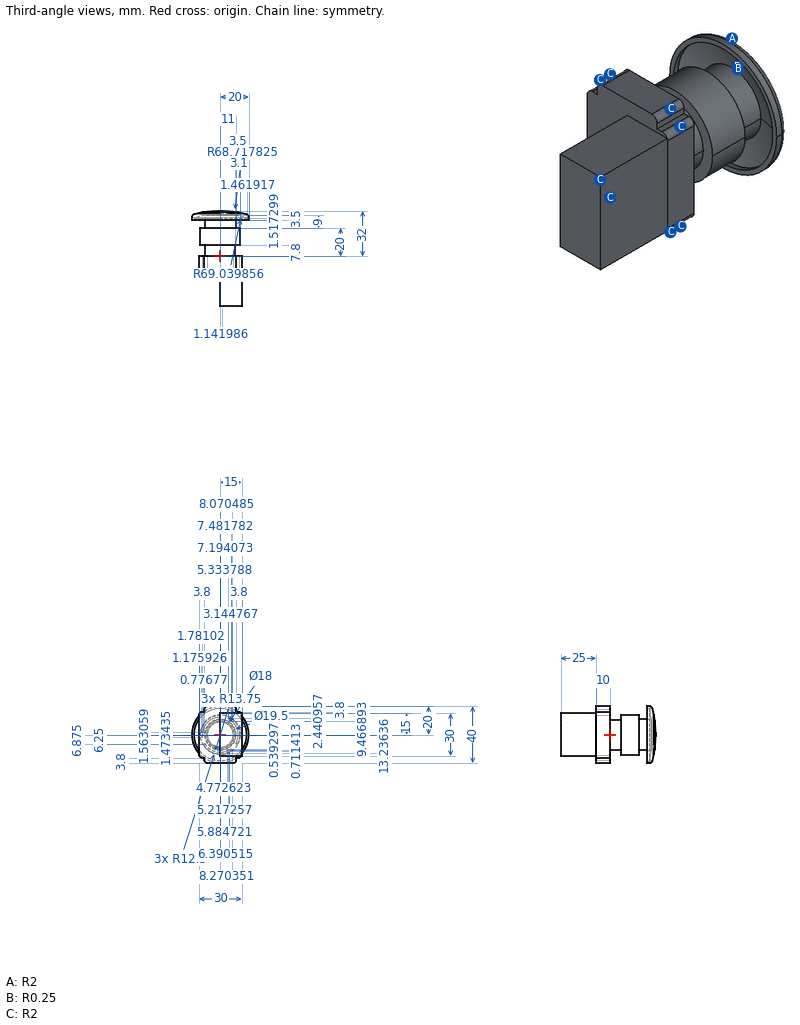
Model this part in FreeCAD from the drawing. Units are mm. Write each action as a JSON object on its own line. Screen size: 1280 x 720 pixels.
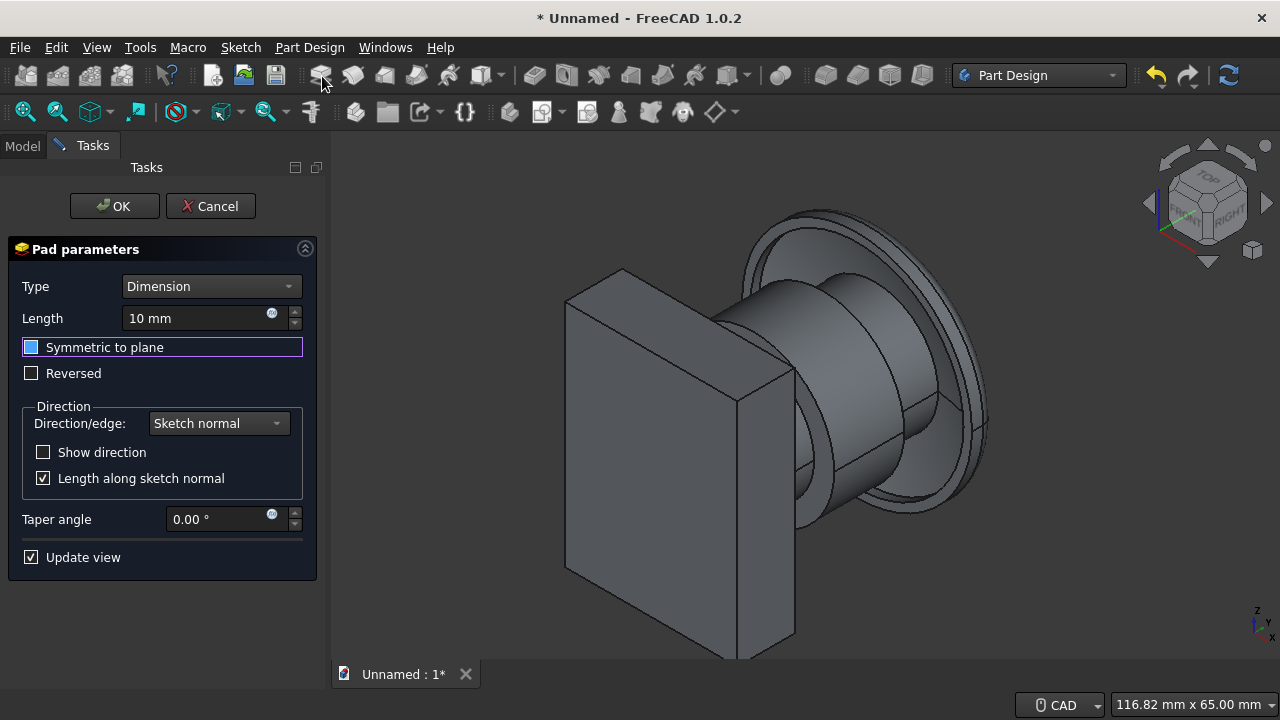
{"action": "left_click", "coordinate": [115, 206]}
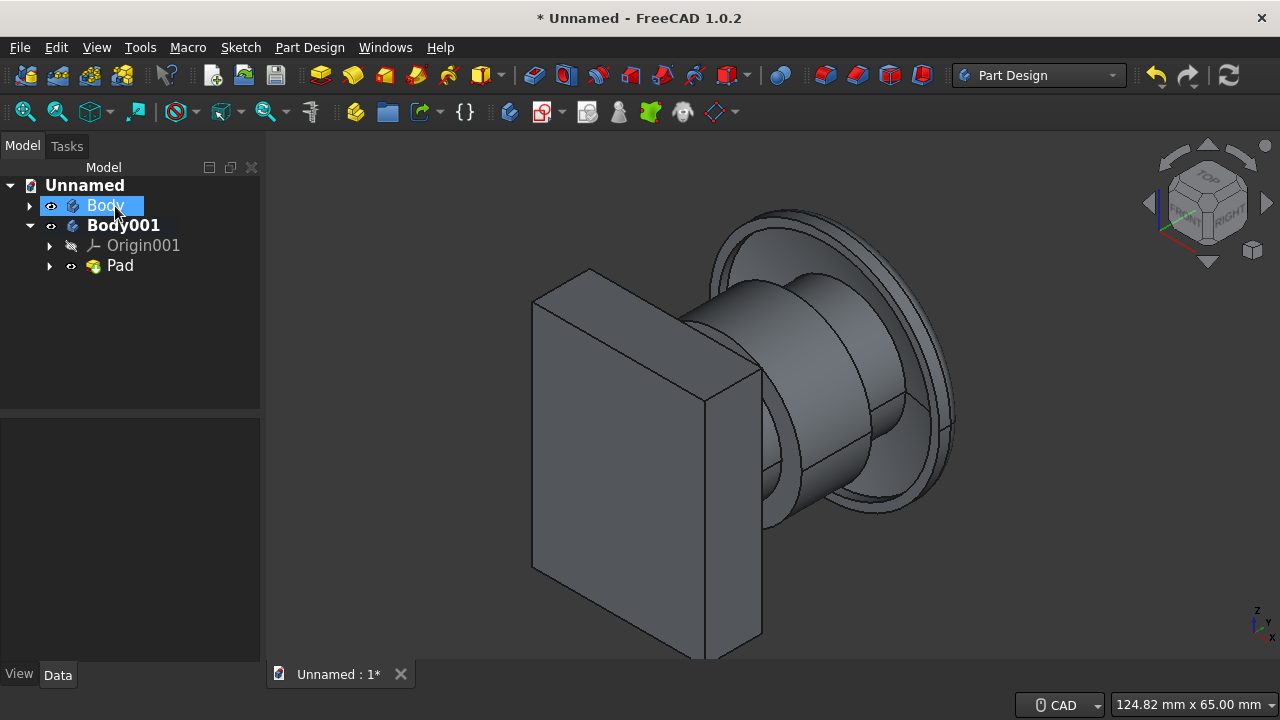
{"action": "left_click", "coordinate": [26, 112]}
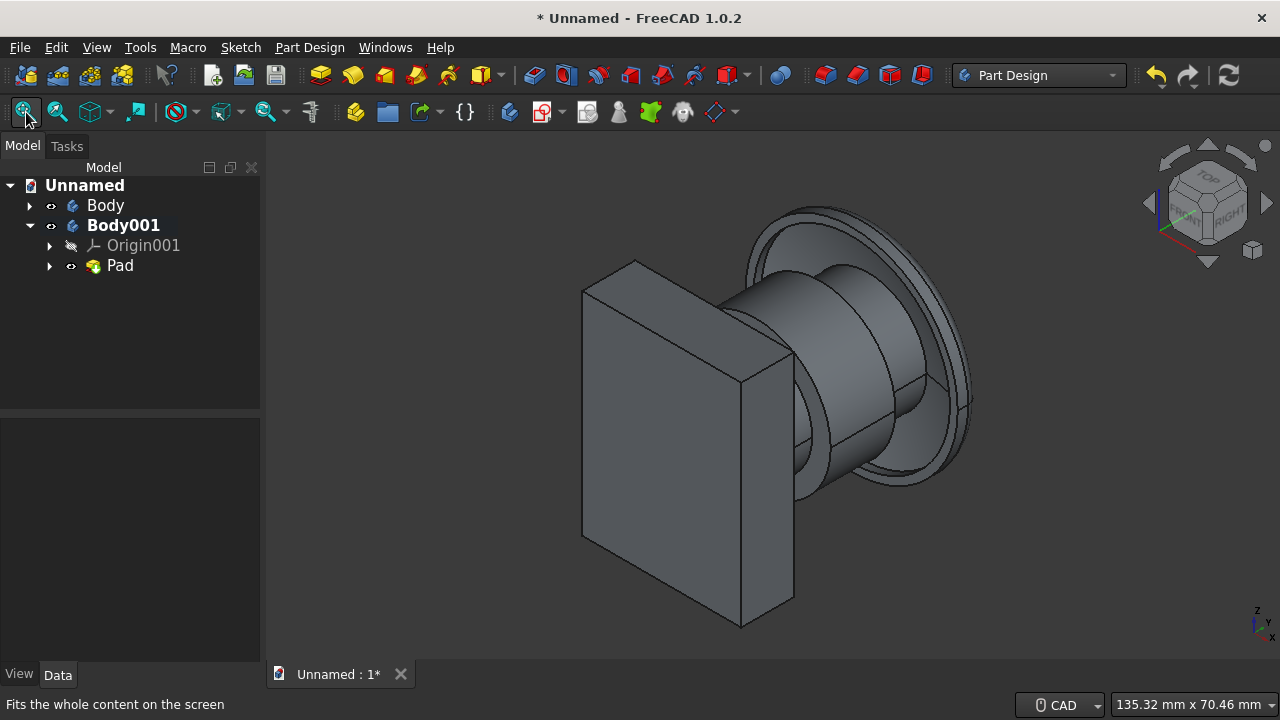
{"action": "left_click", "coordinate": [542, 112]}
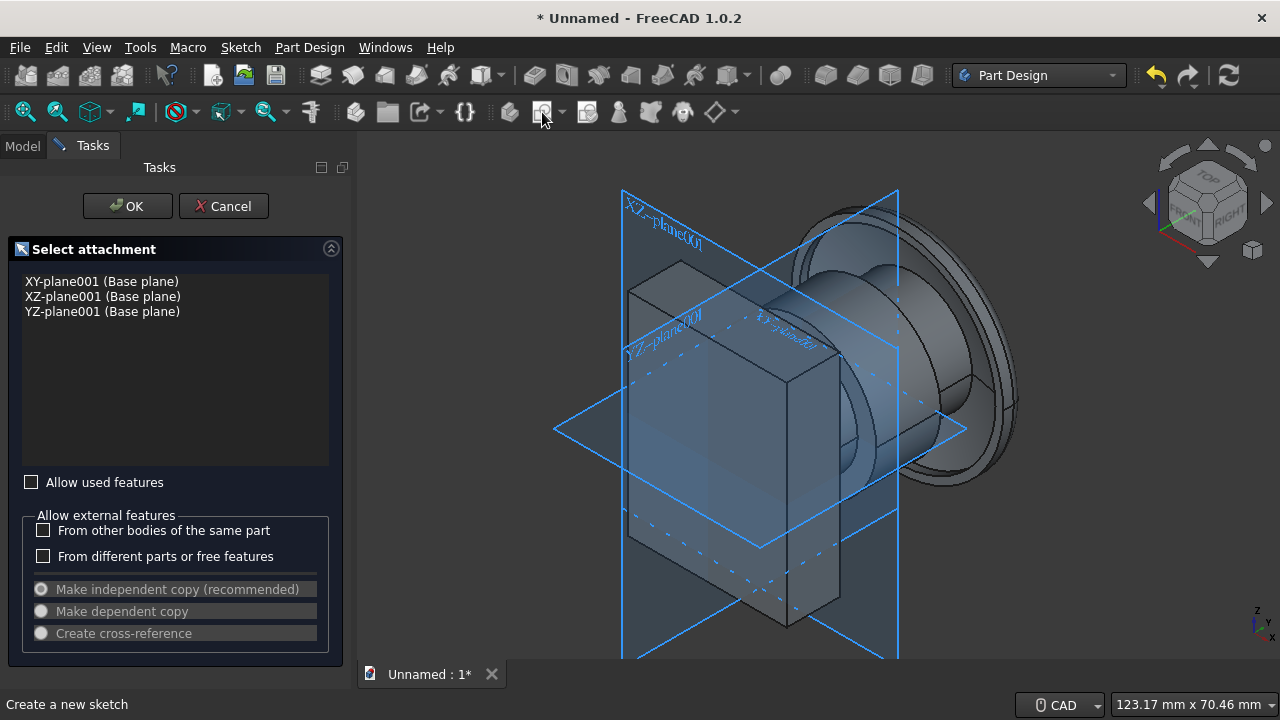
{"action": "left_click", "coordinate": [82, 296]}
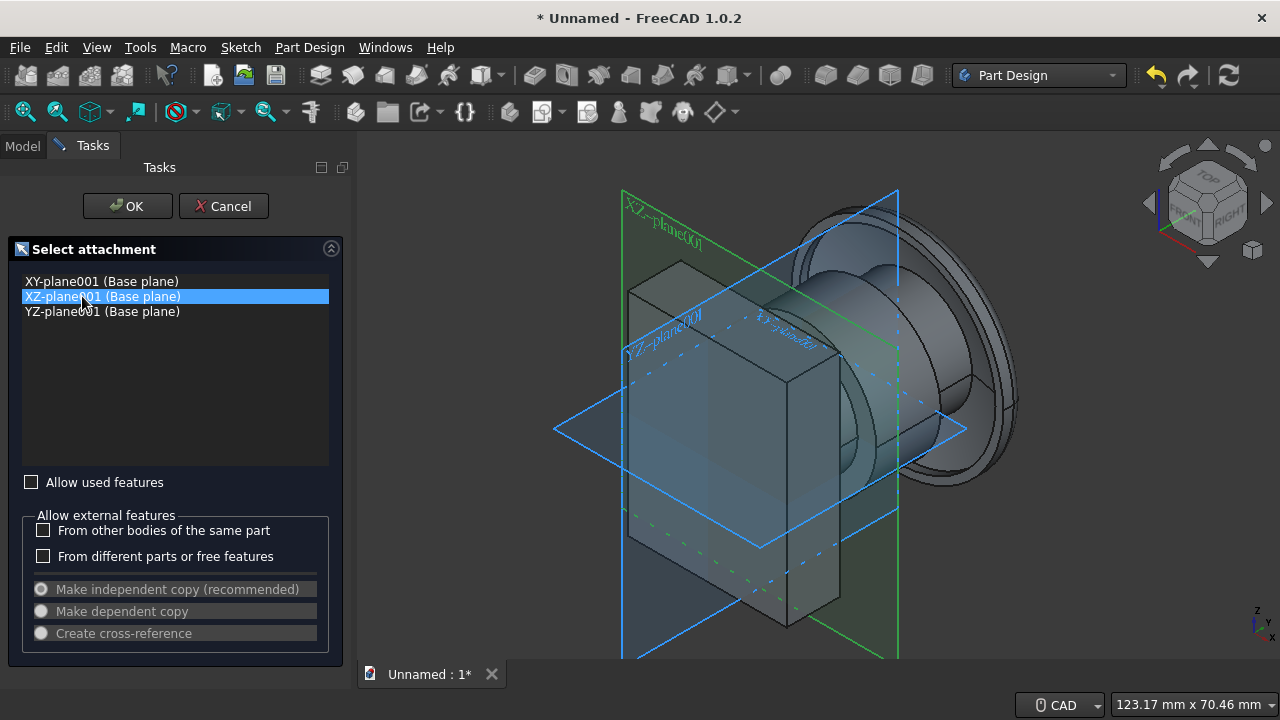
{"action": "left_click", "coordinate": [128, 206]}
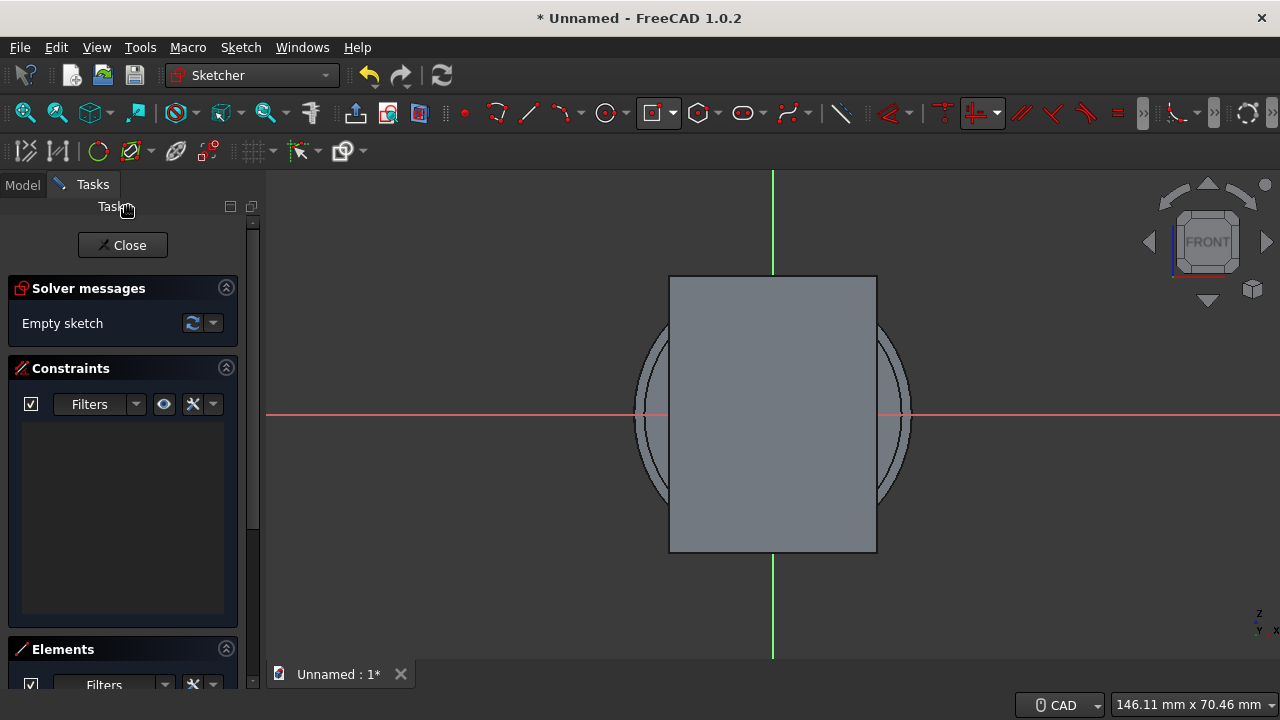
{"action": "left_click", "coordinate": [420, 114]}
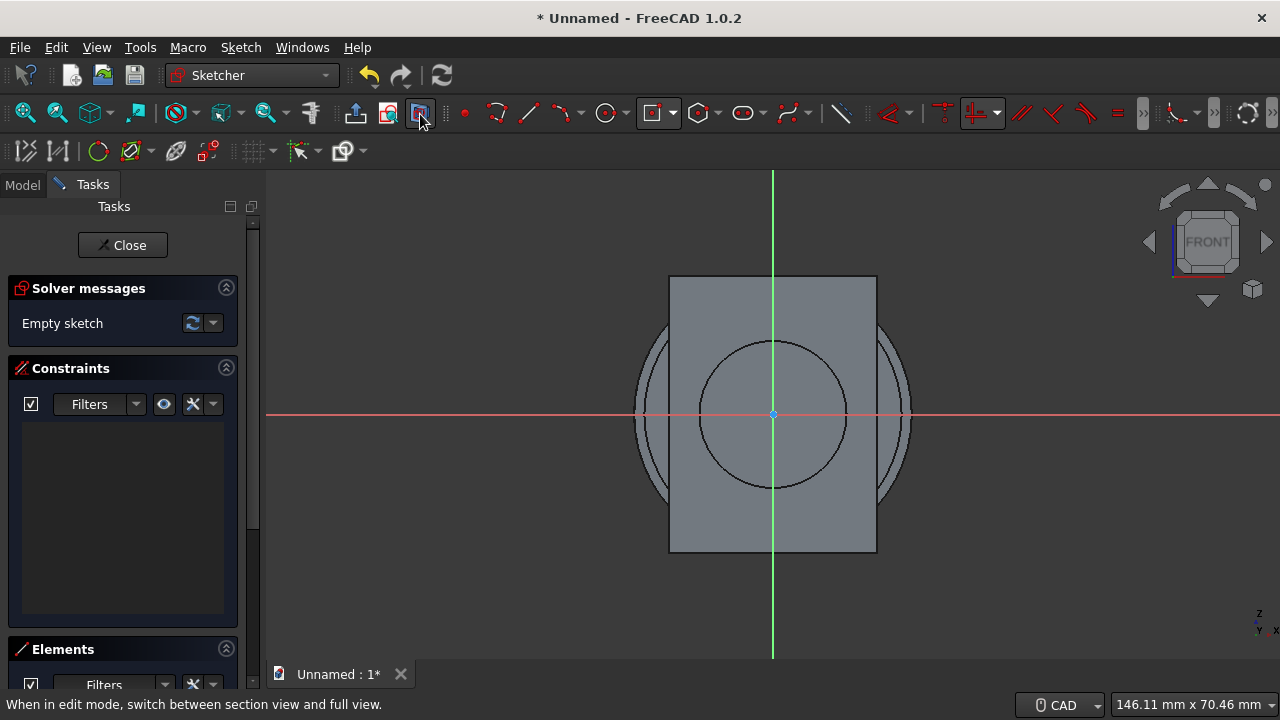
{"action": "left_click", "coordinate": [676, 114]}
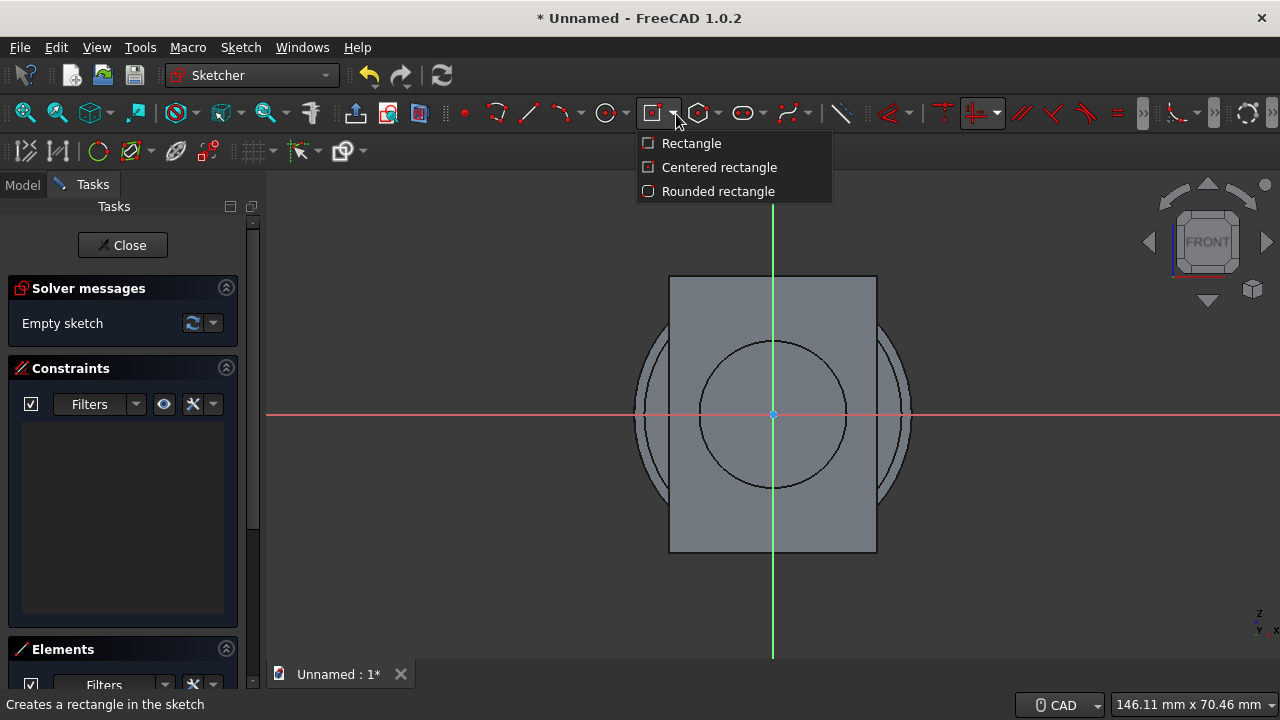
{"action": "left_click", "coordinate": [734, 143]}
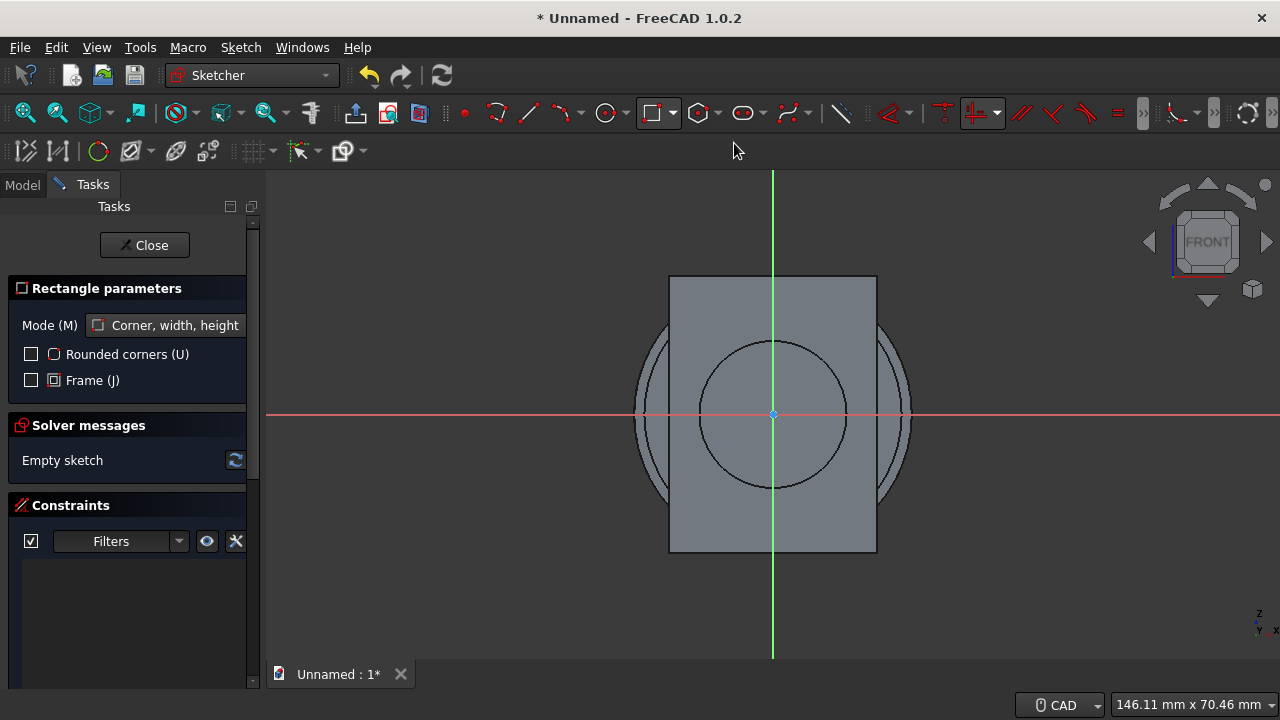
{"action": "left_click", "coordinate": [851, 276]}
{"action": "mouse_move", "coordinate": [877, 302]}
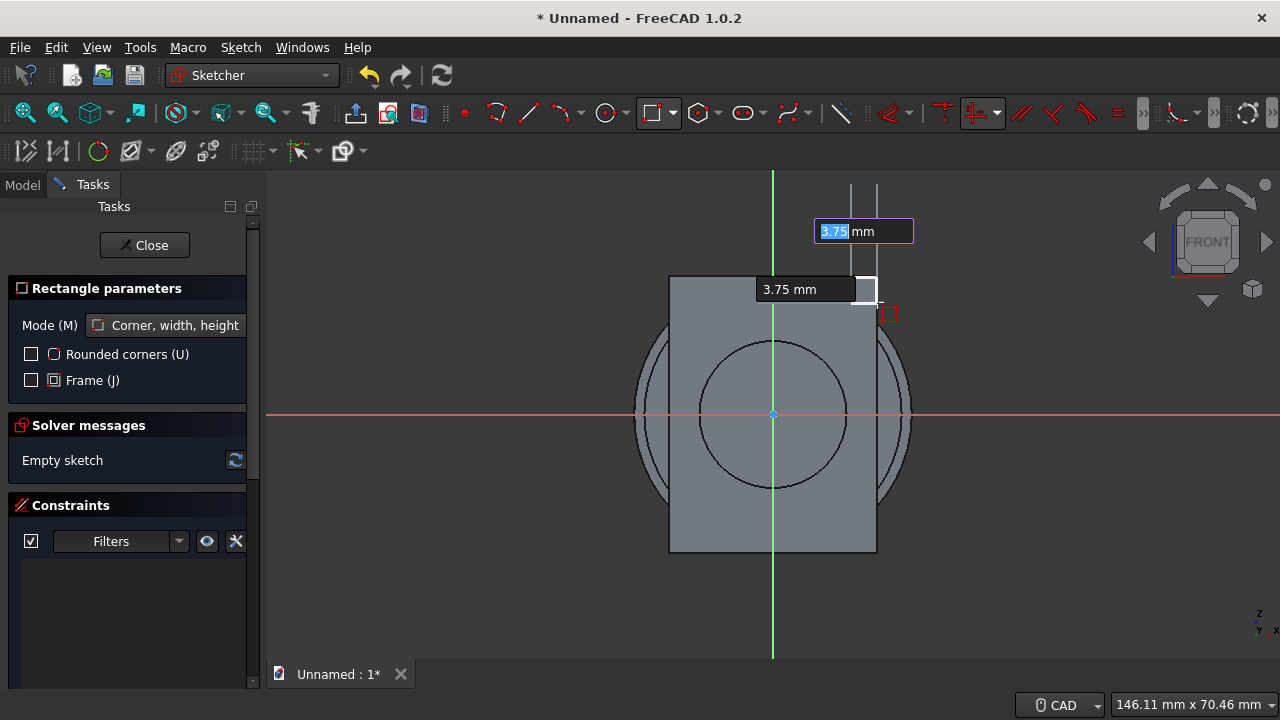
{"action": "type", "text": "3.8"}
{"action": "key", "text": "Tab"}
{"action": "type", "text": "3.8"}
{"action": "key", "text": "Return"}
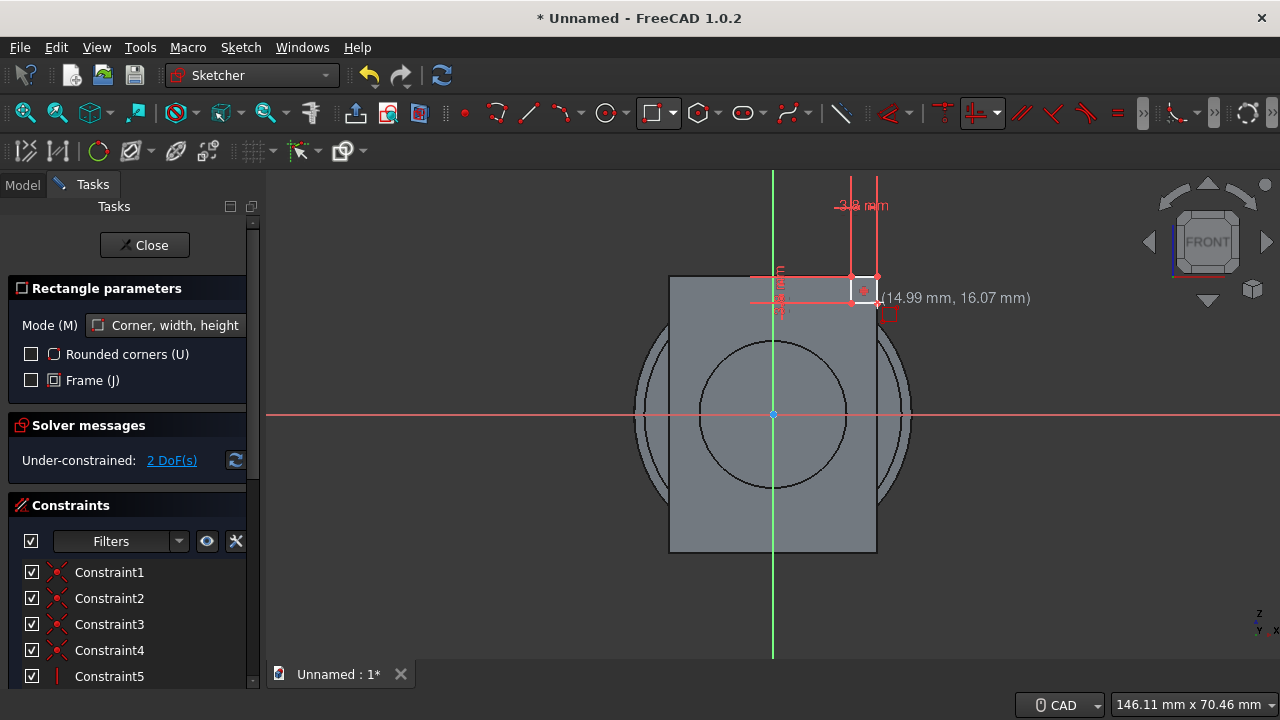
{"action": "left_click", "coordinate": [669, 276]}
{"action": "mouse_move", "coordinate": [695, 302]}